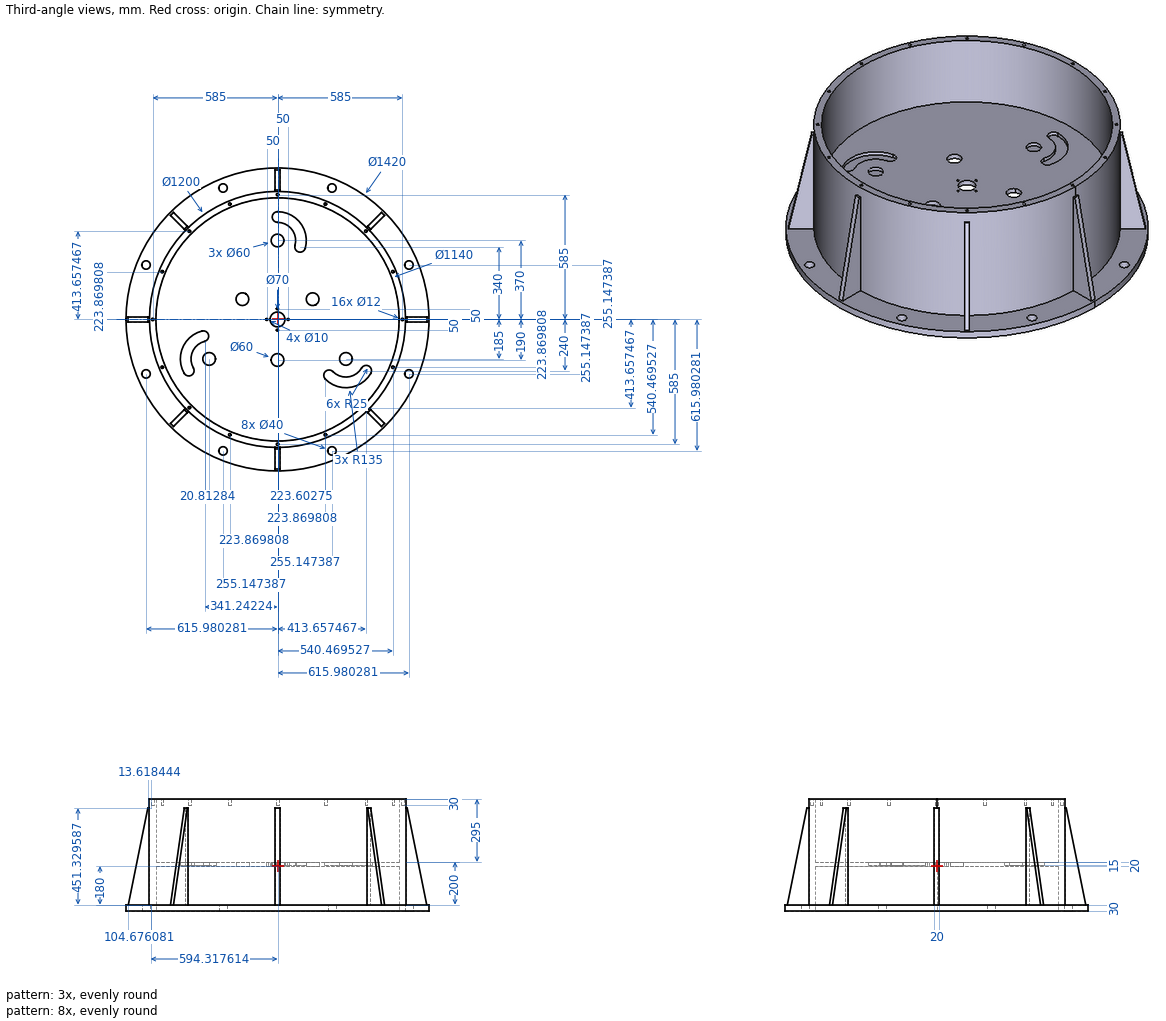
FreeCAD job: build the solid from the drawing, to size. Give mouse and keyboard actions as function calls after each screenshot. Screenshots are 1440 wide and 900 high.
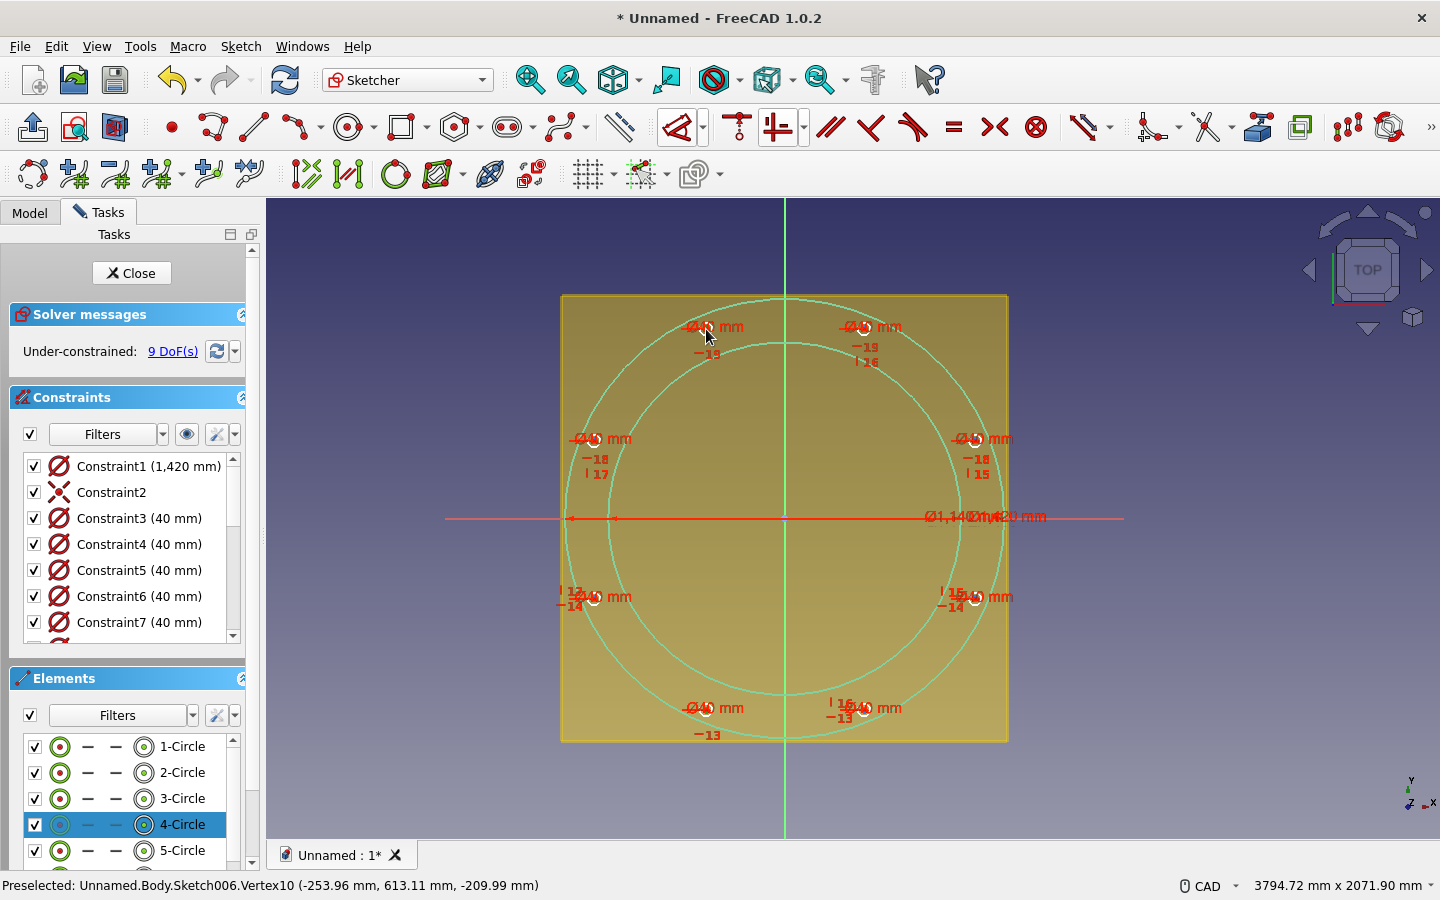
click(504, 519)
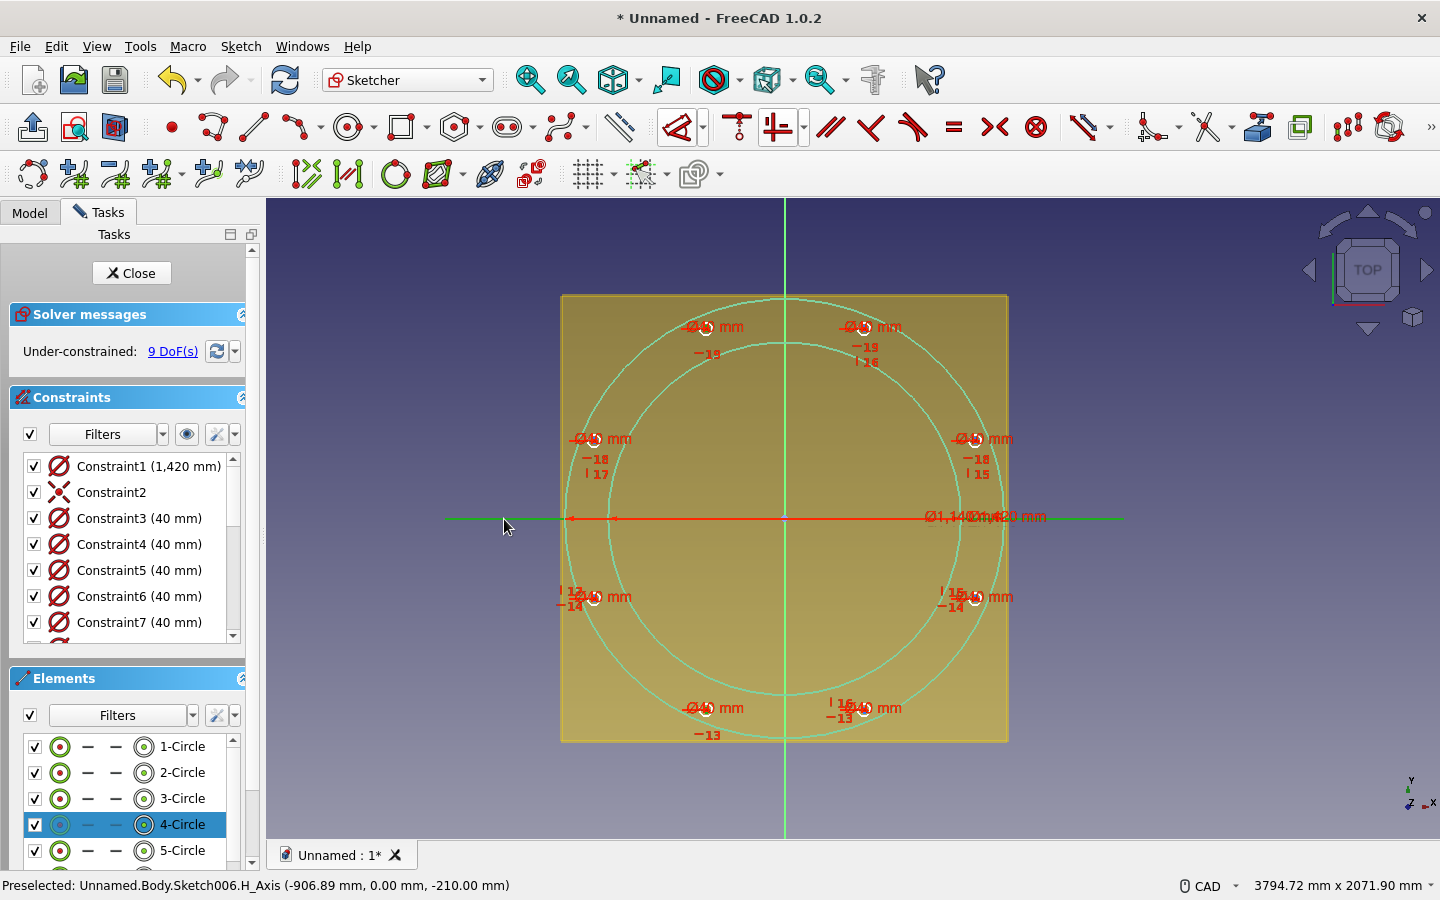
key(s)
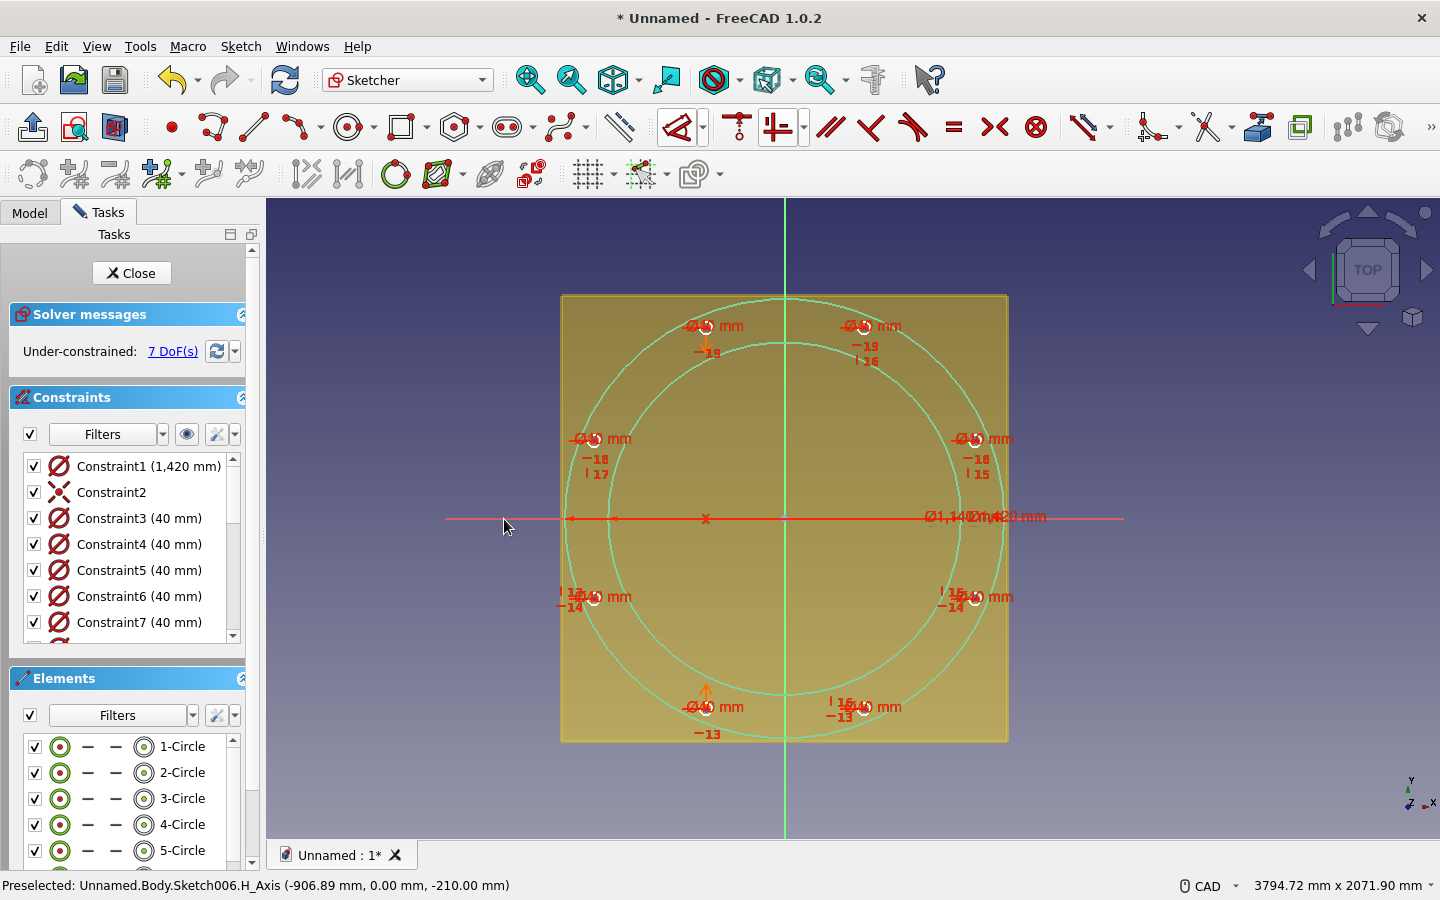
click(864, 709)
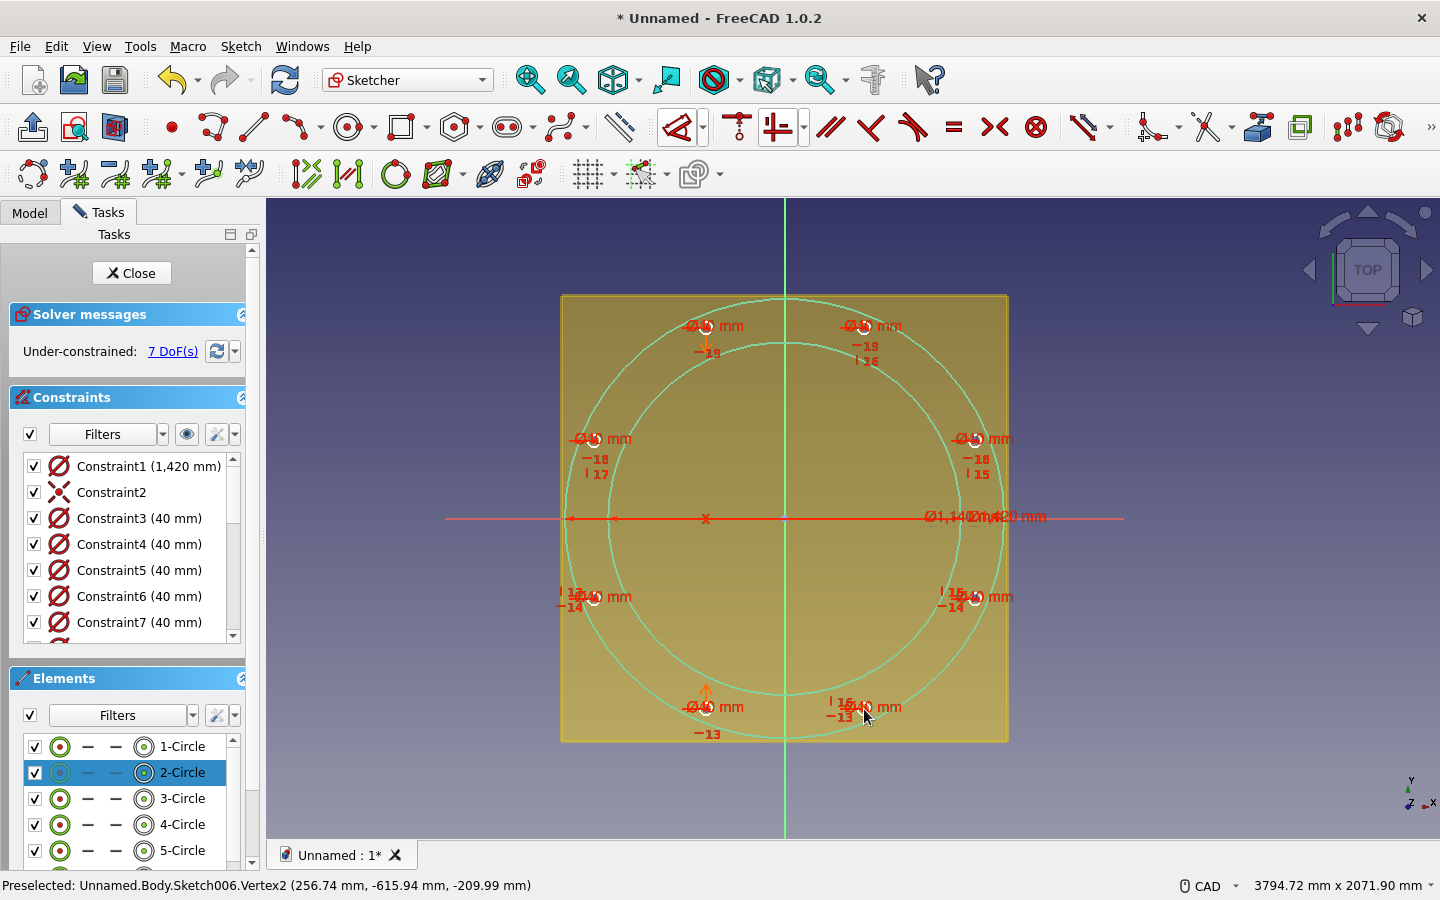
click(702, 128)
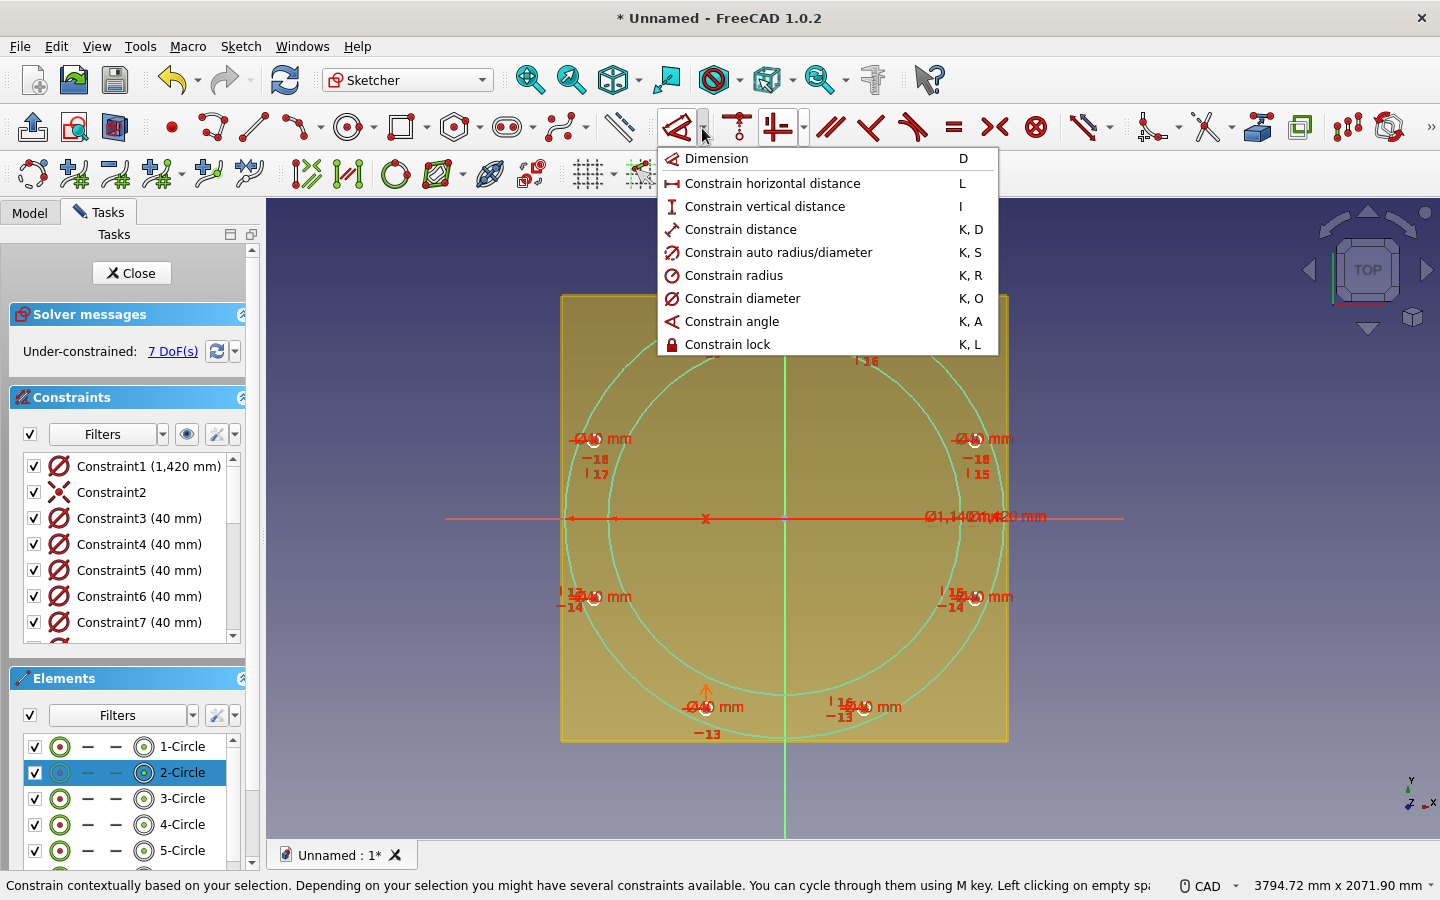
click(828, 184)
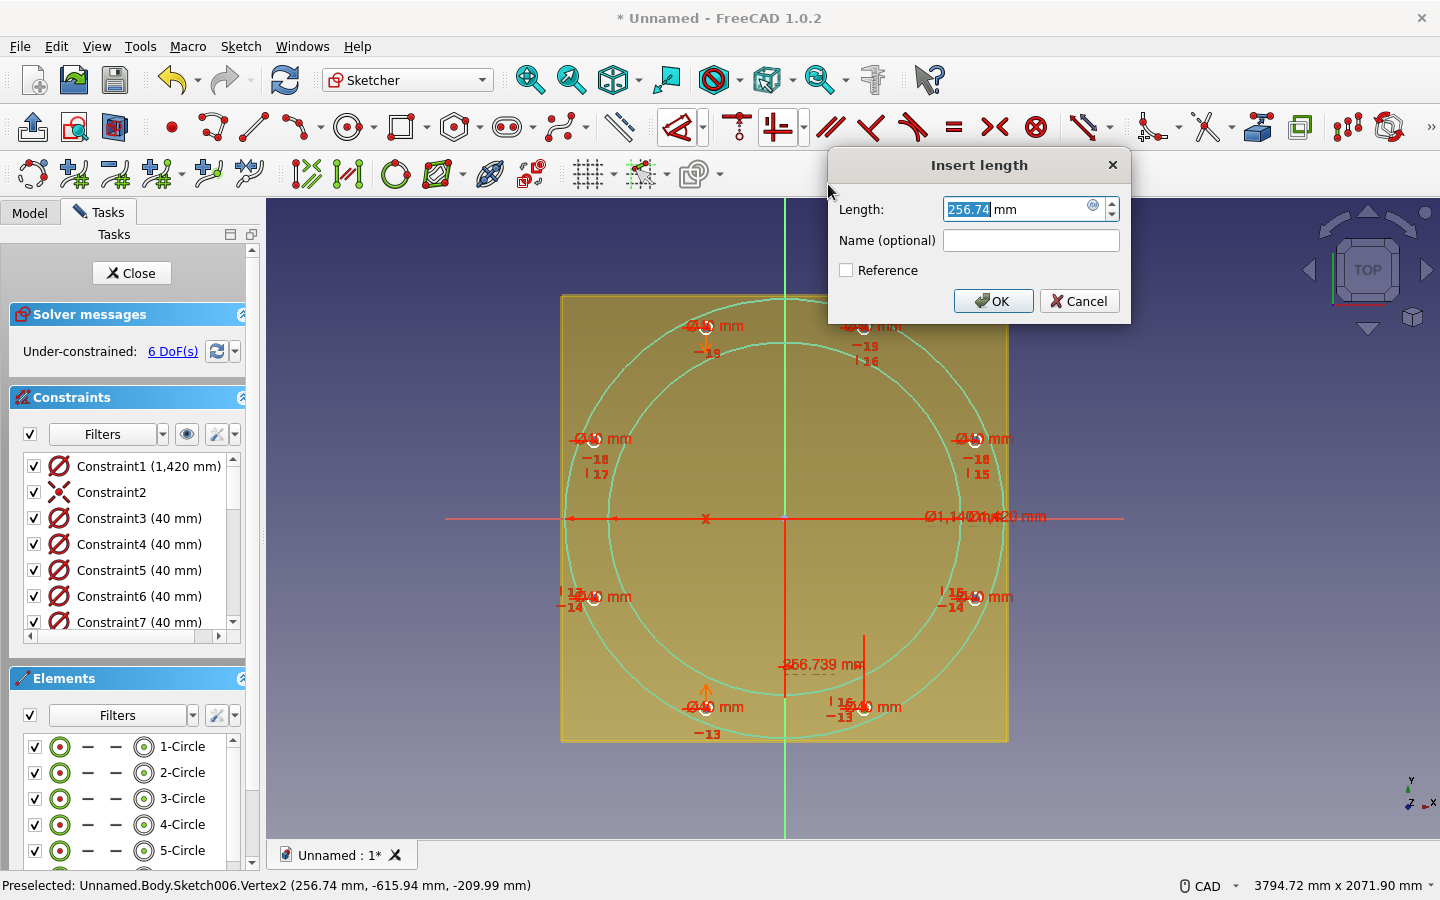
text(255.147387)
key(Return)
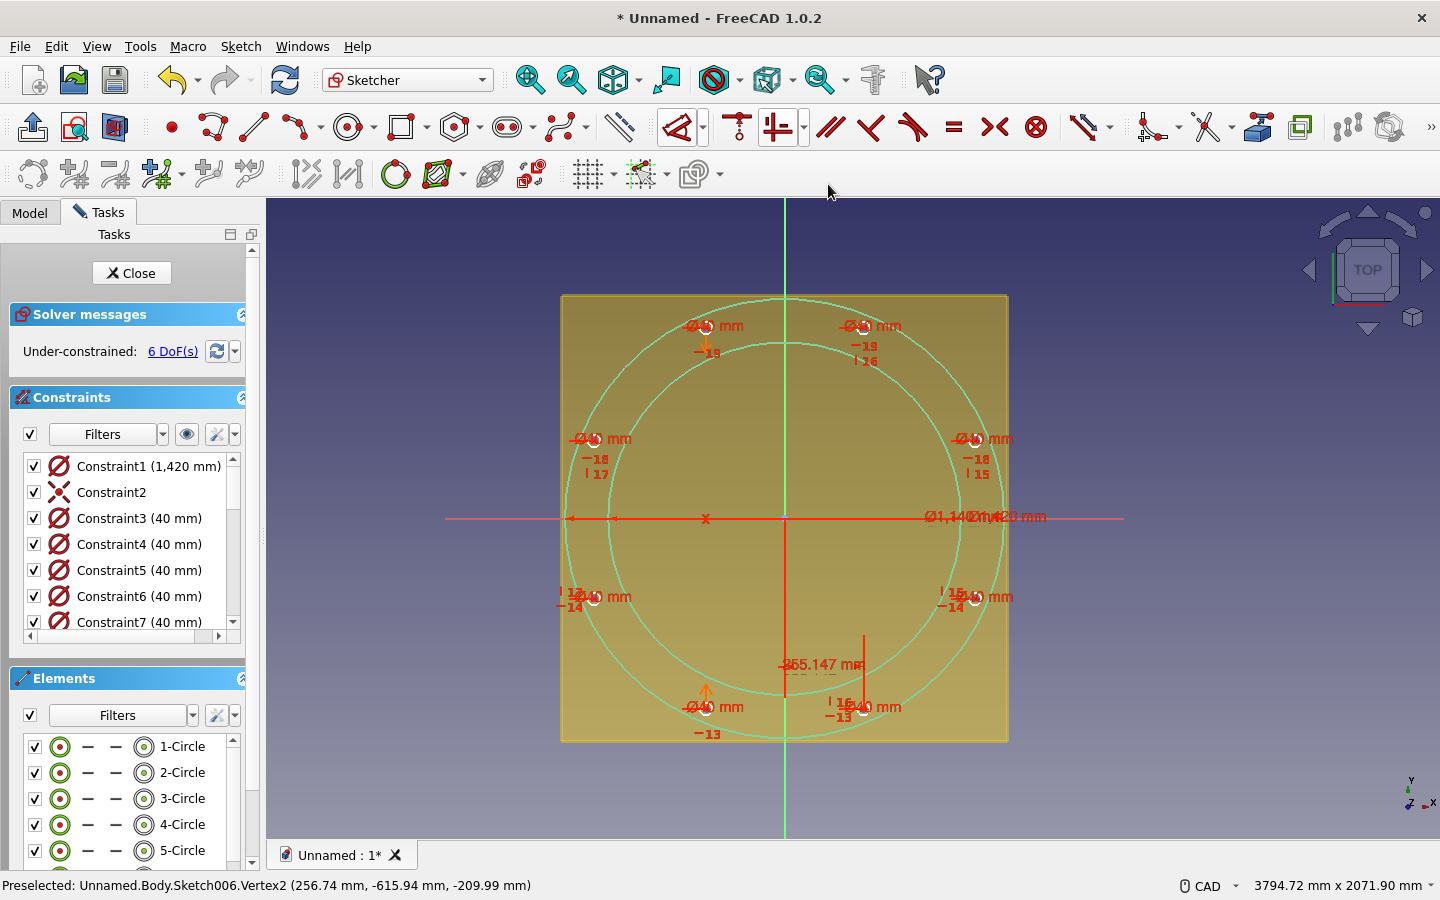
click(864, 709)